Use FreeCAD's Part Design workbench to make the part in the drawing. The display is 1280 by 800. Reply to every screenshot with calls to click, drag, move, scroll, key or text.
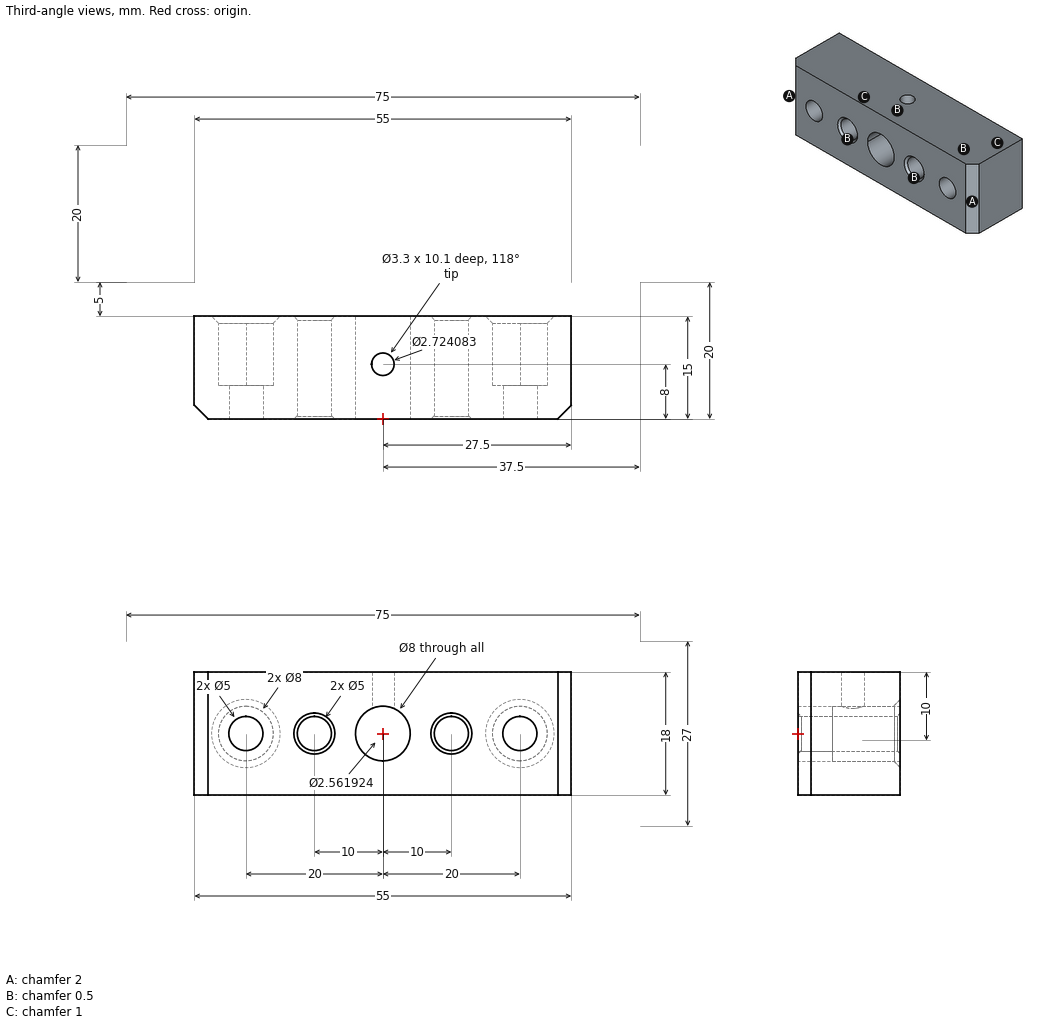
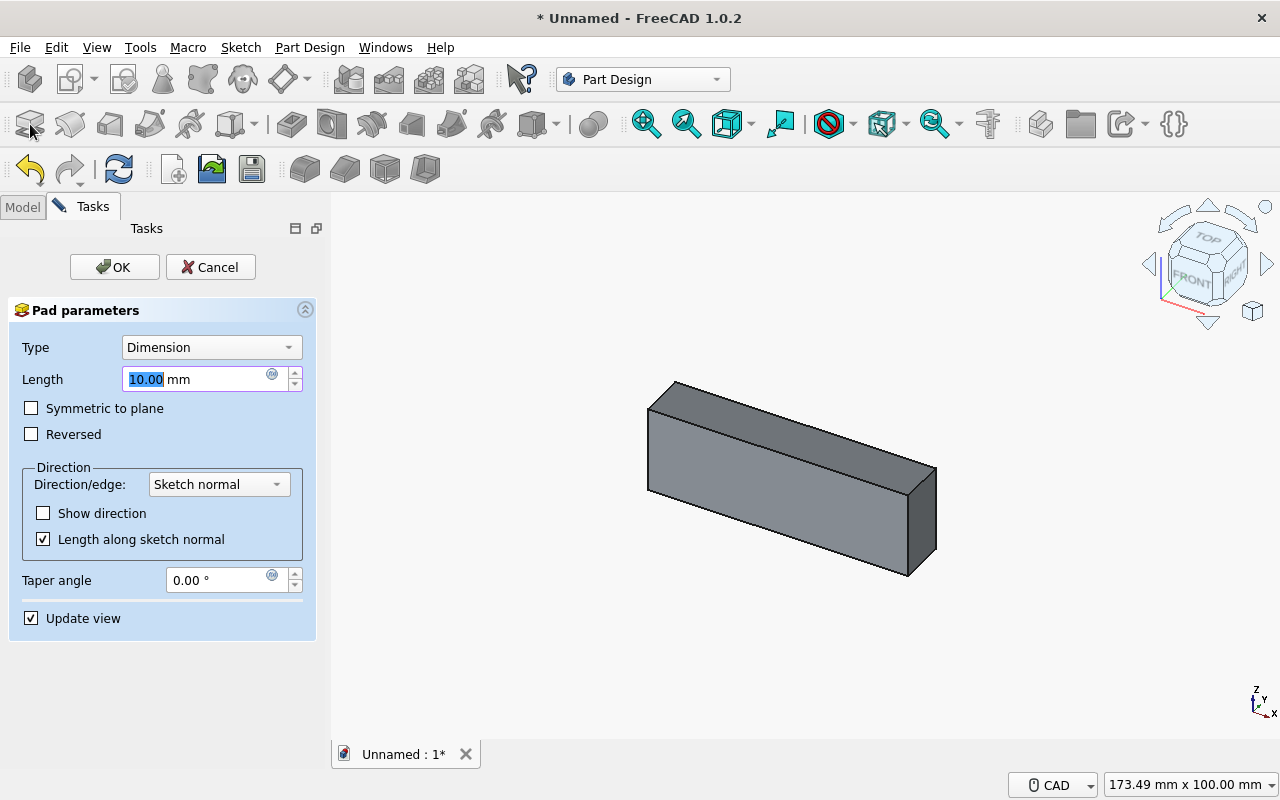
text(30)
key(Tab)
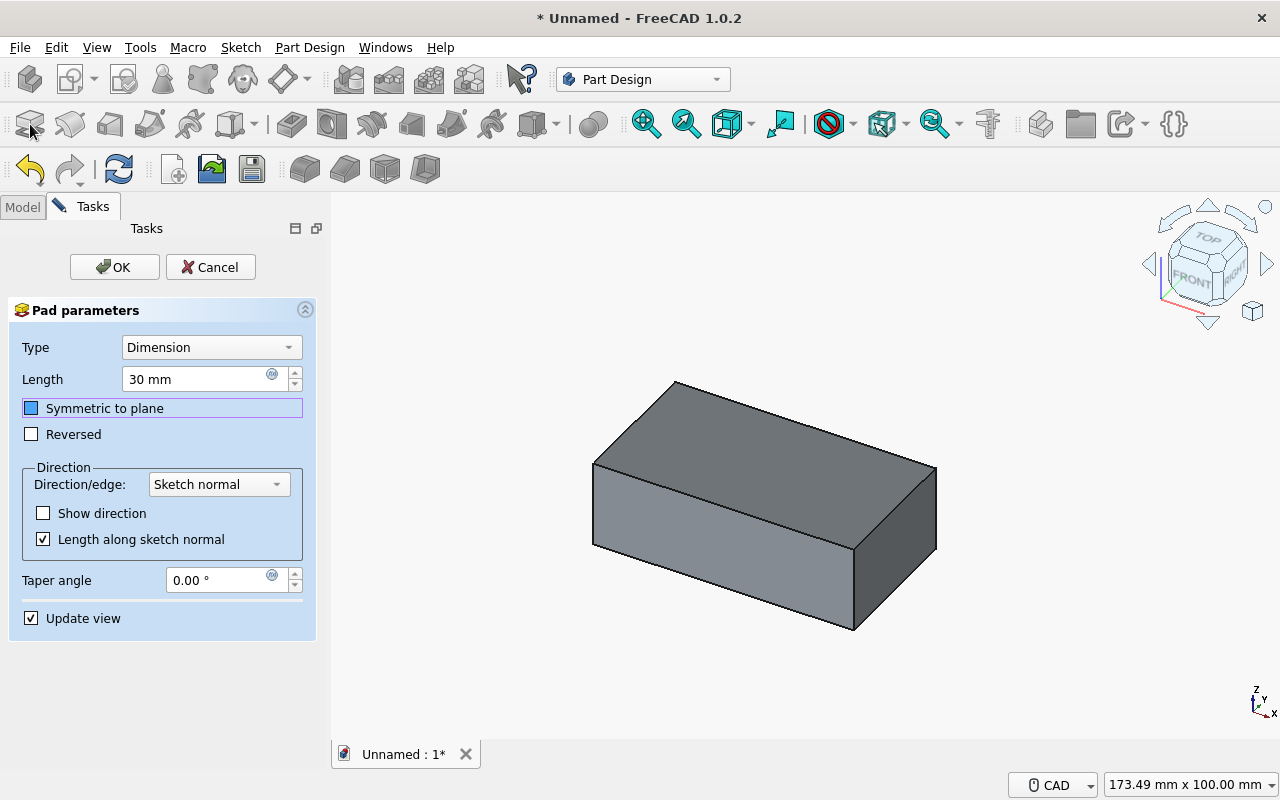
click(30, 434)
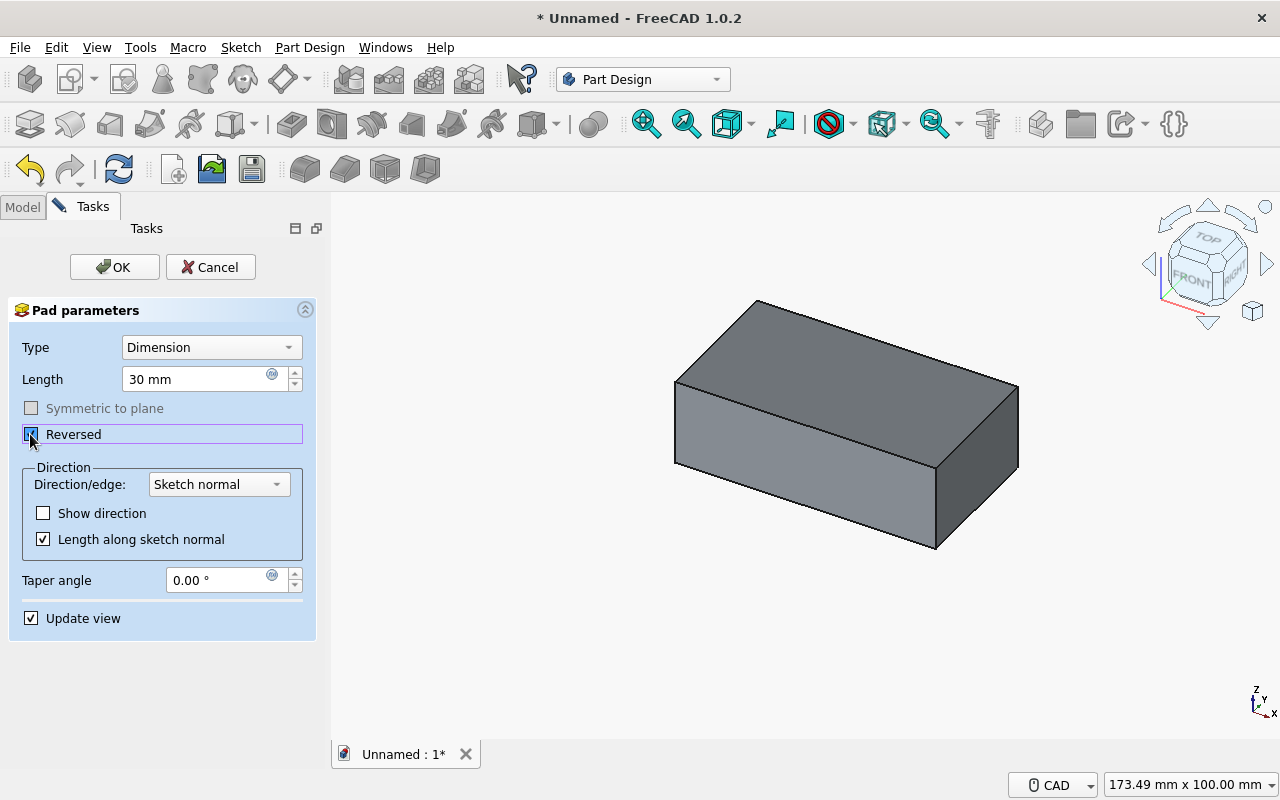
click(115, 267)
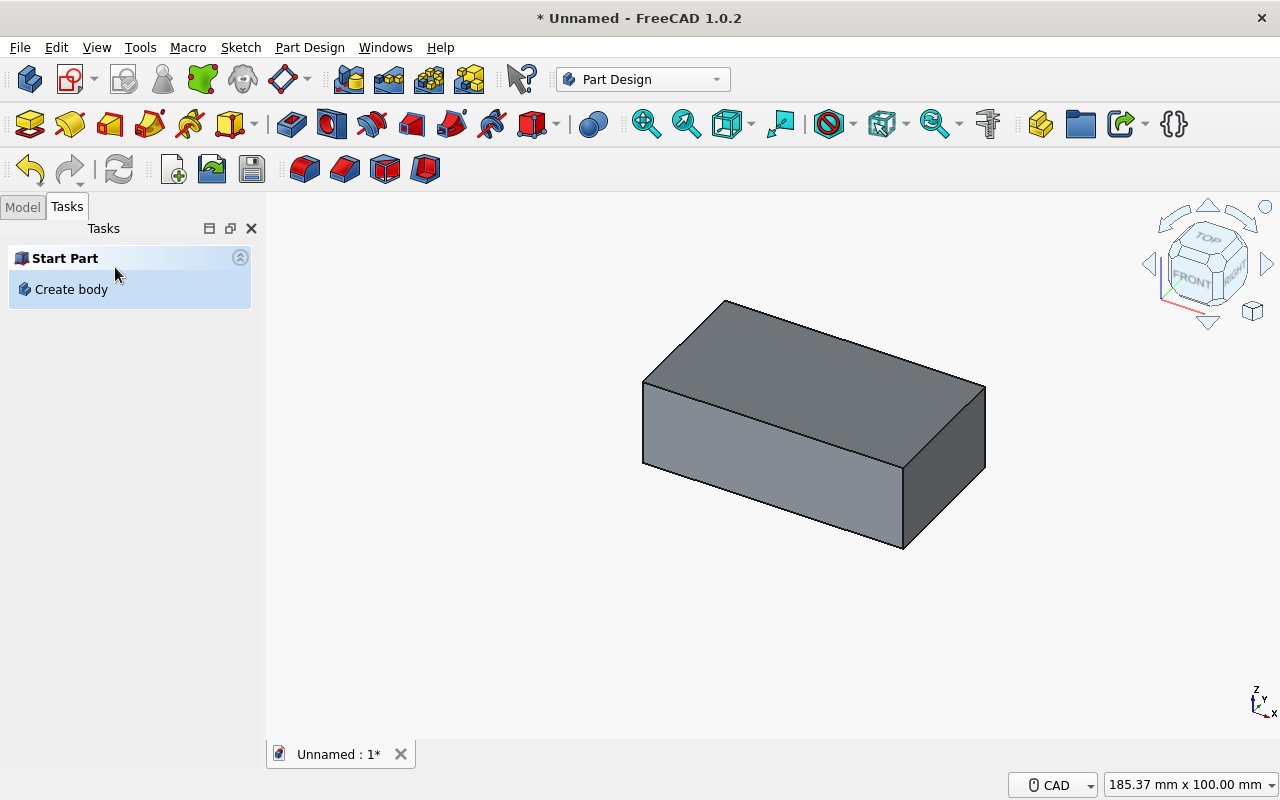
key(4)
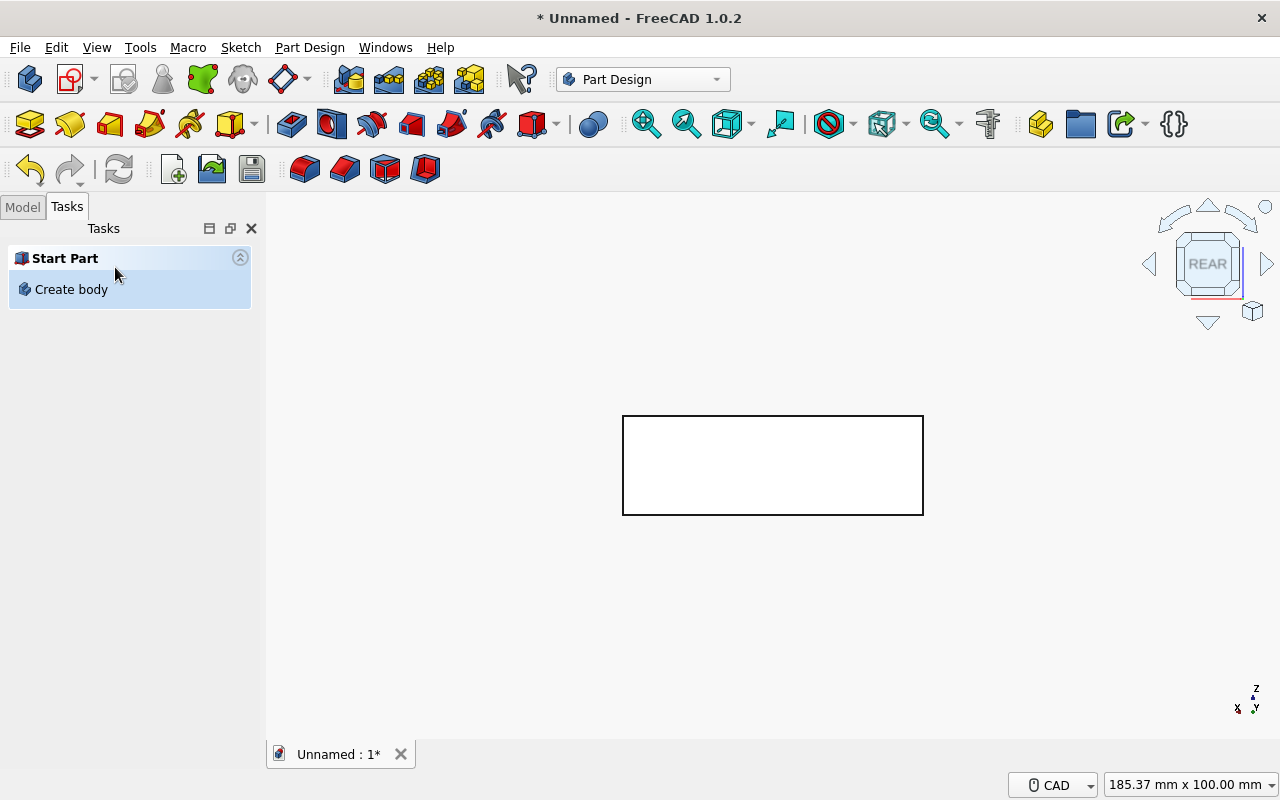
click(648, 124)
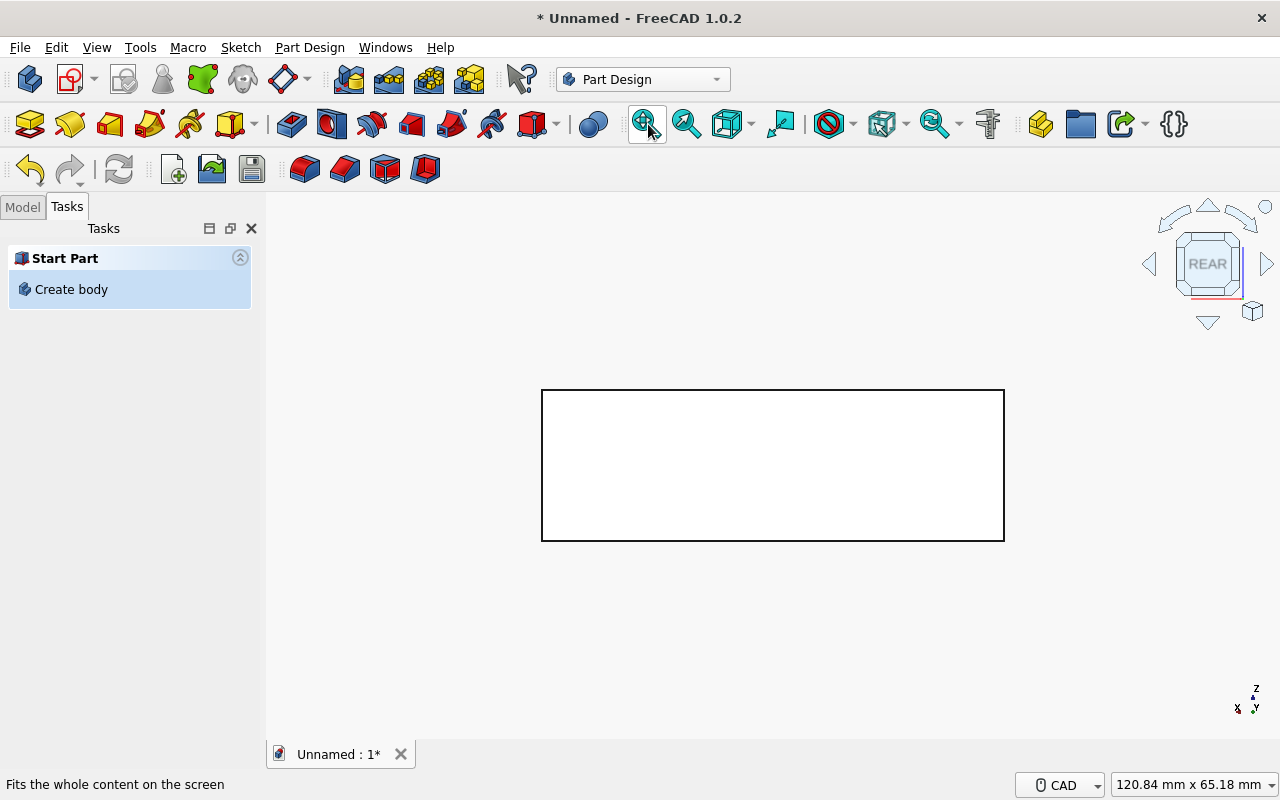
click(641, 465)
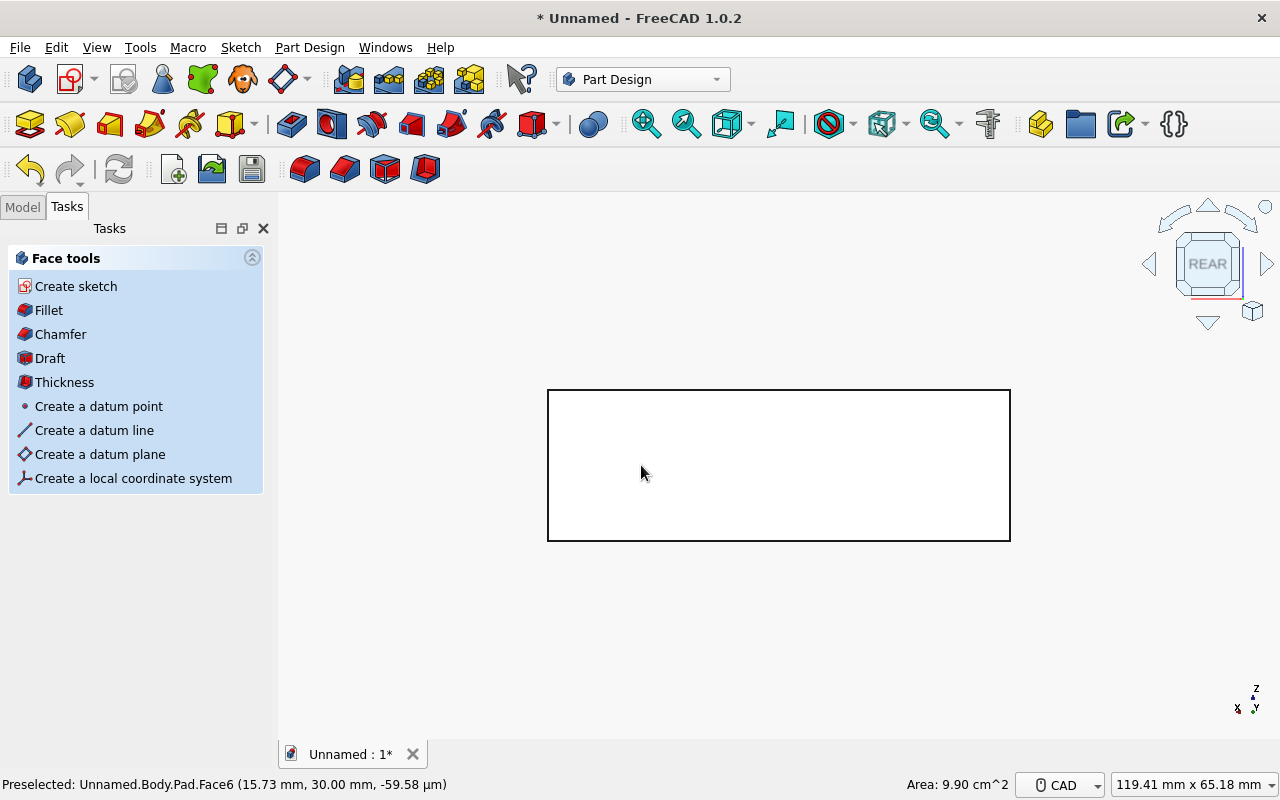
click(70, 80)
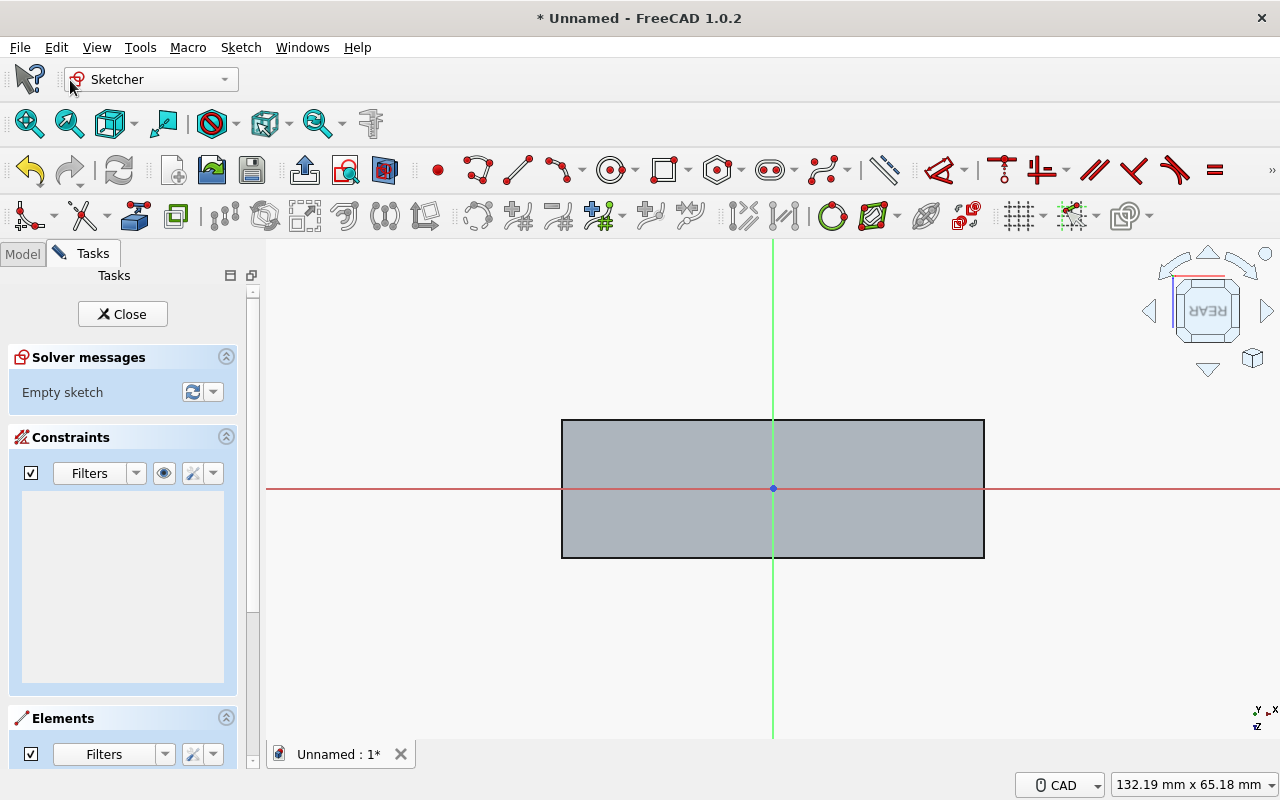
scroll(912, 489, up, 2)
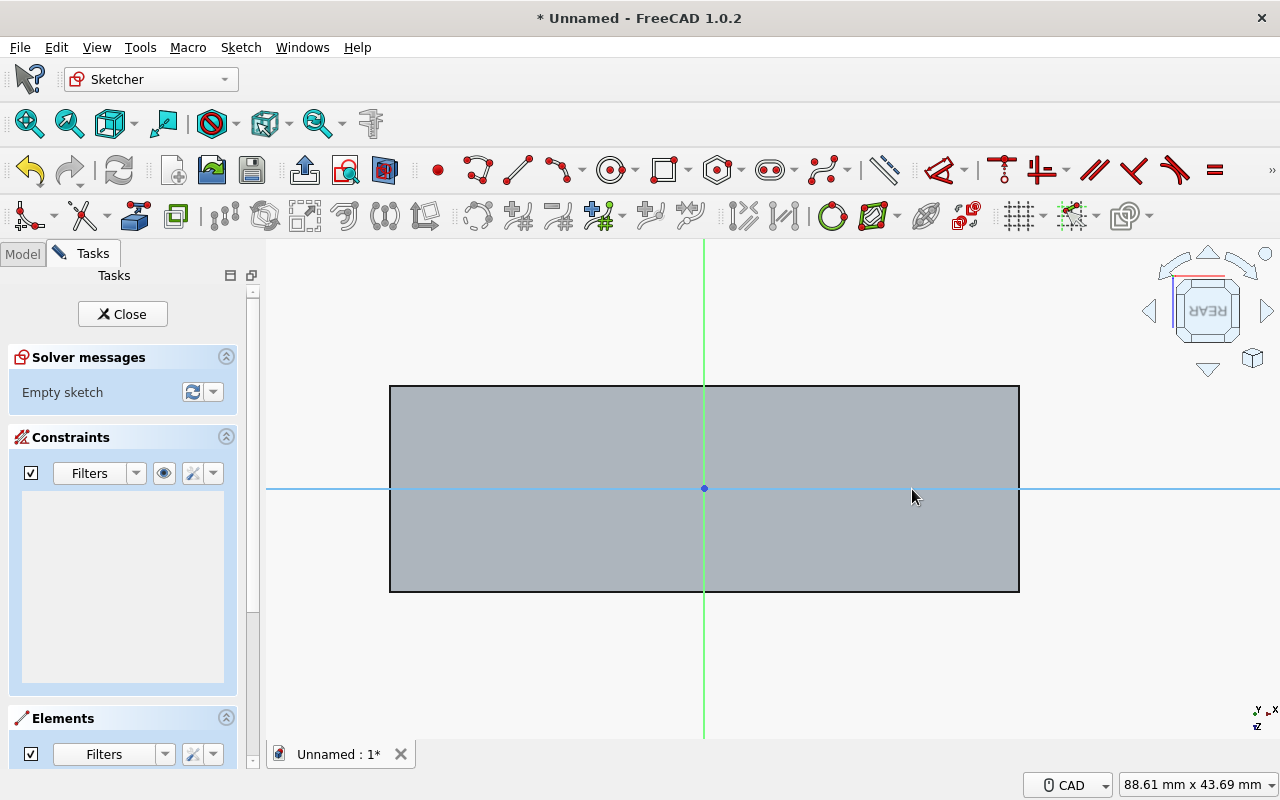
click(612, 170)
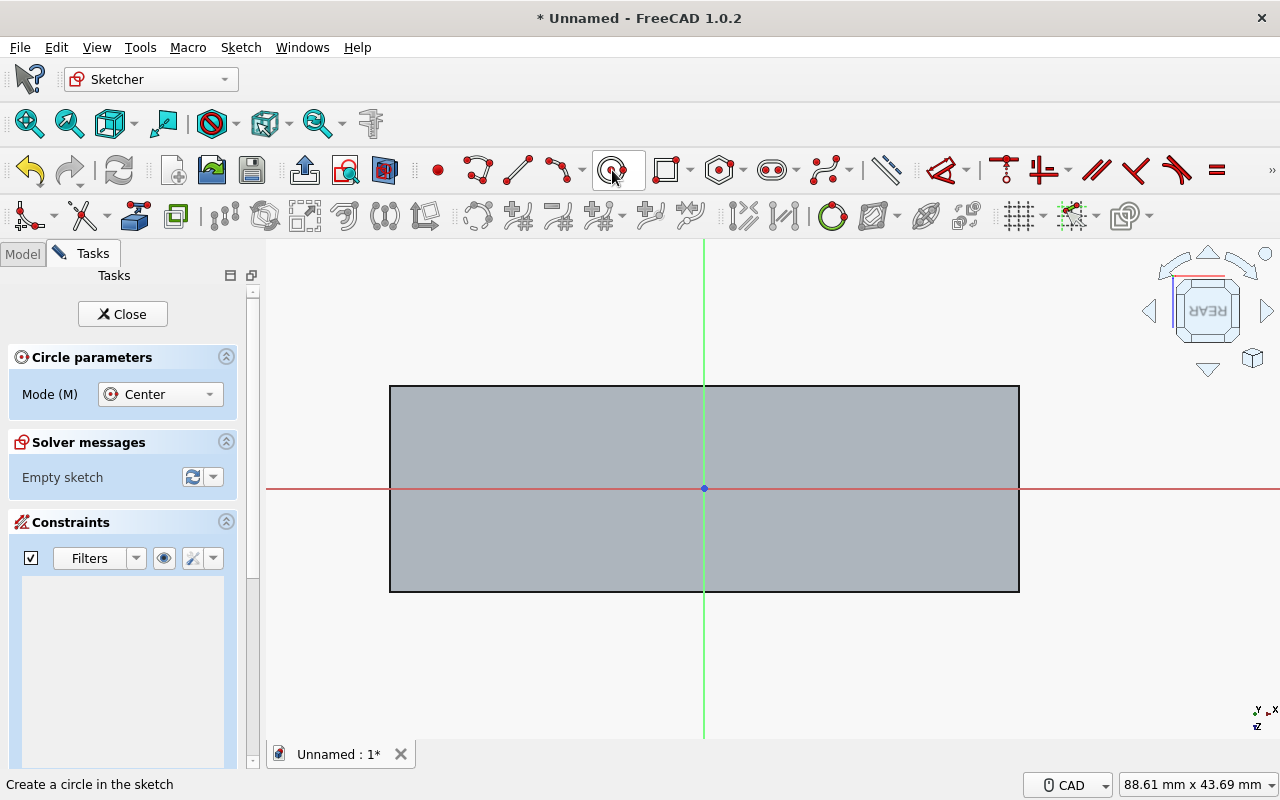
click(475, 489)
move(508, 456)